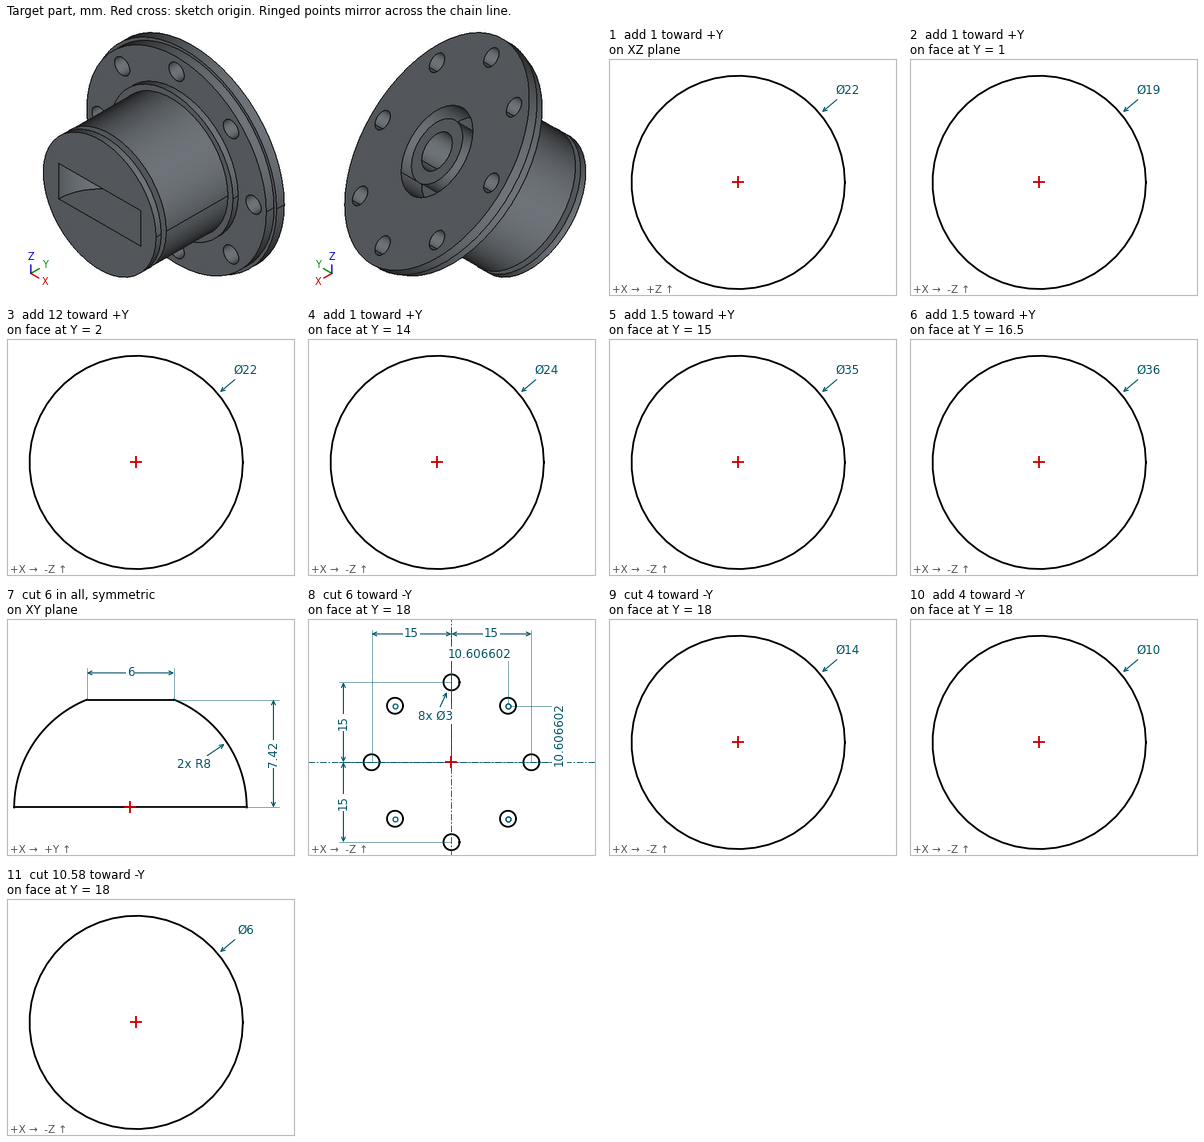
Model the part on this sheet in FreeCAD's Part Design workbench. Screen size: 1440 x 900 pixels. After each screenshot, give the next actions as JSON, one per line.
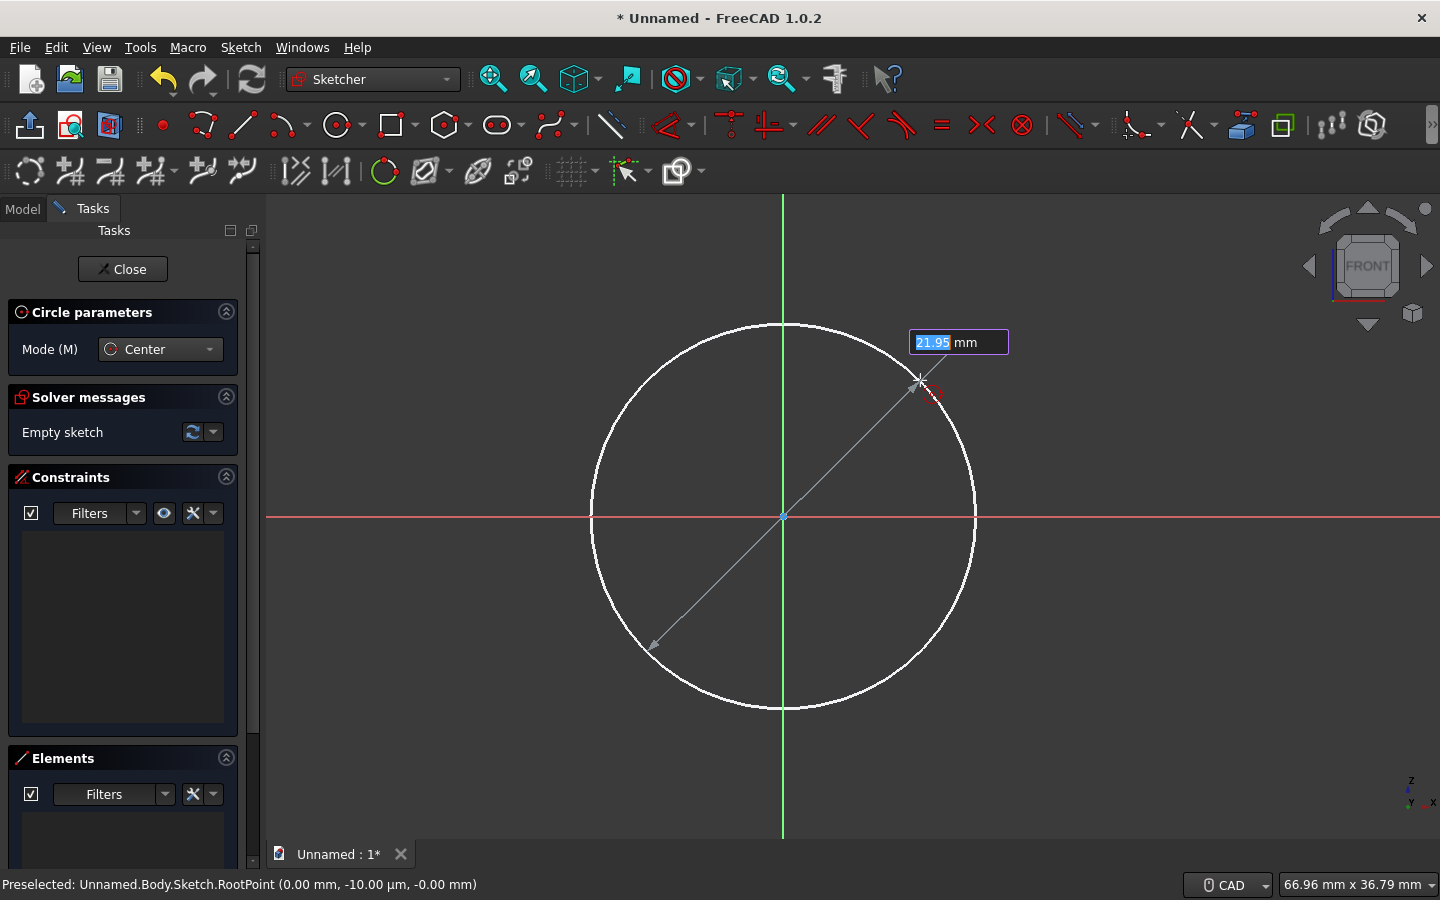
{"action": "type", "text": "22"}
{"action": "key", "text": "Return"}
{"action": "key", "text": "Escape"}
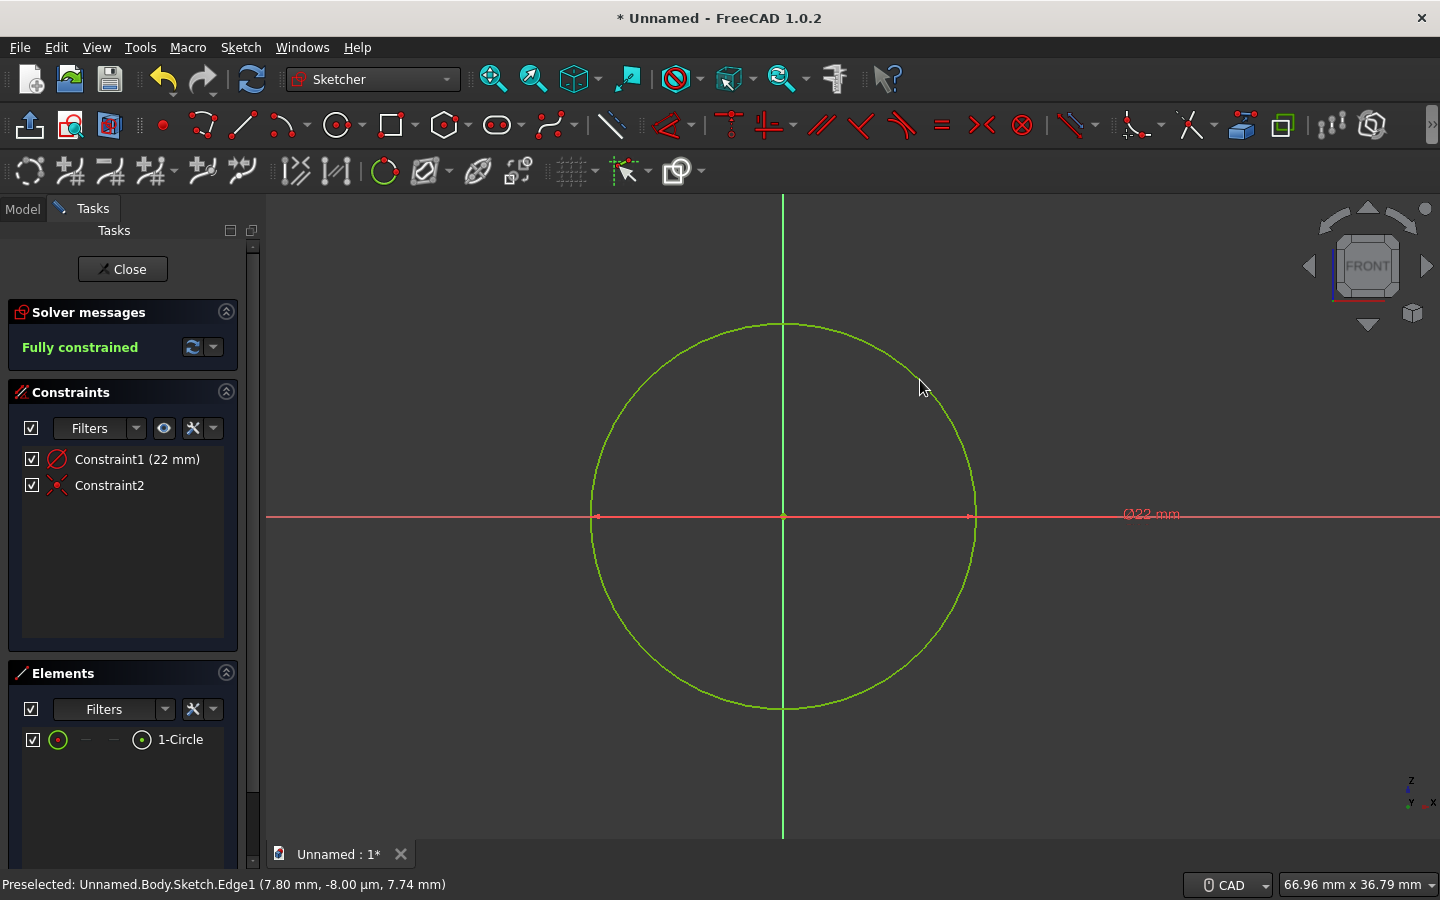
{"action": "left_click", "coordinate": [123, 269]}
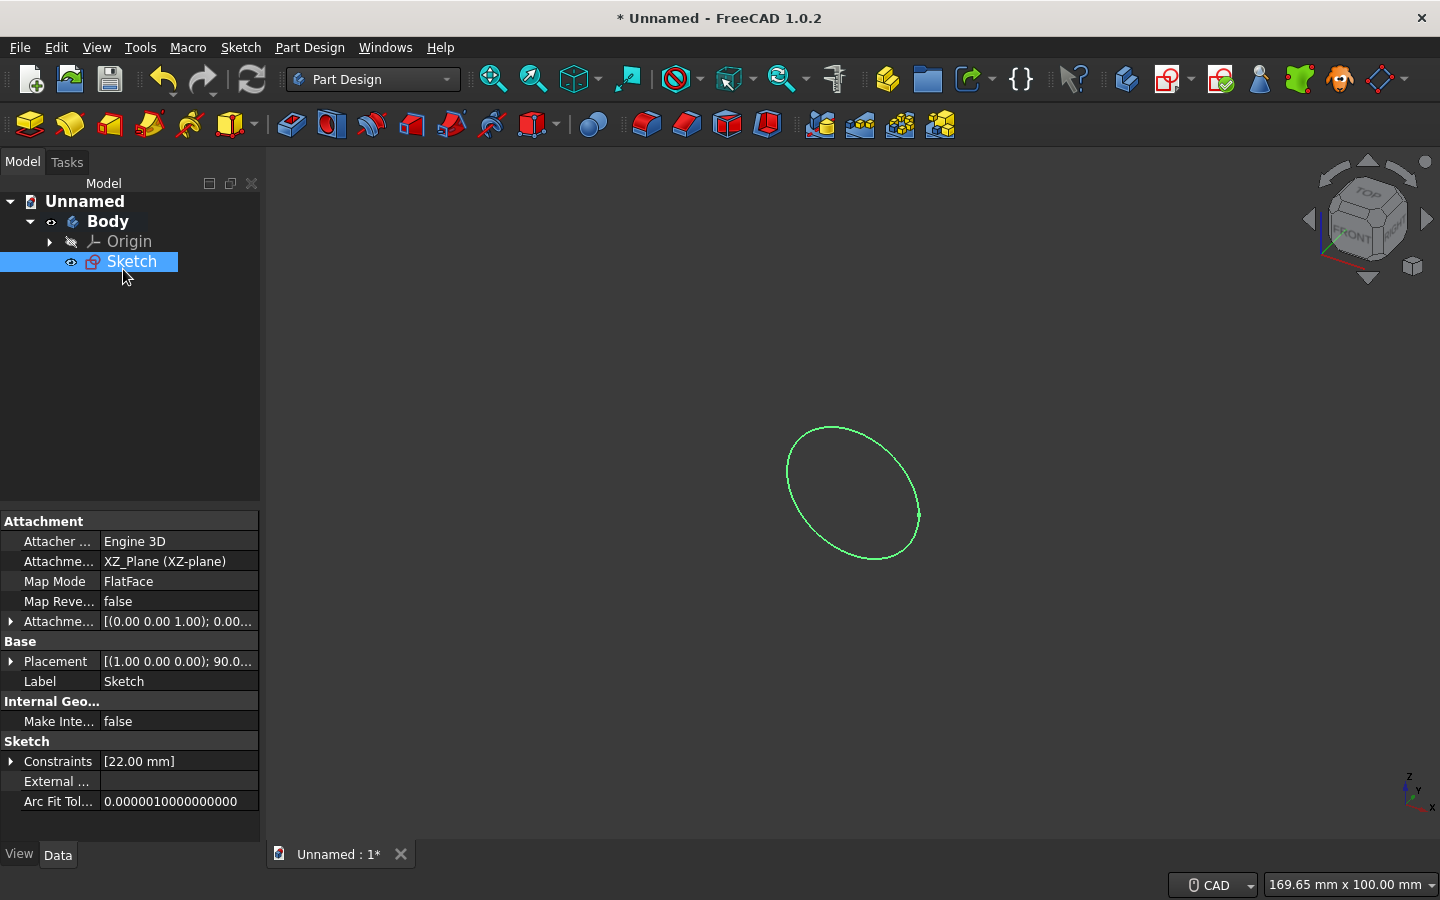
{"action": "left_click", "coordinate": [30, 124]}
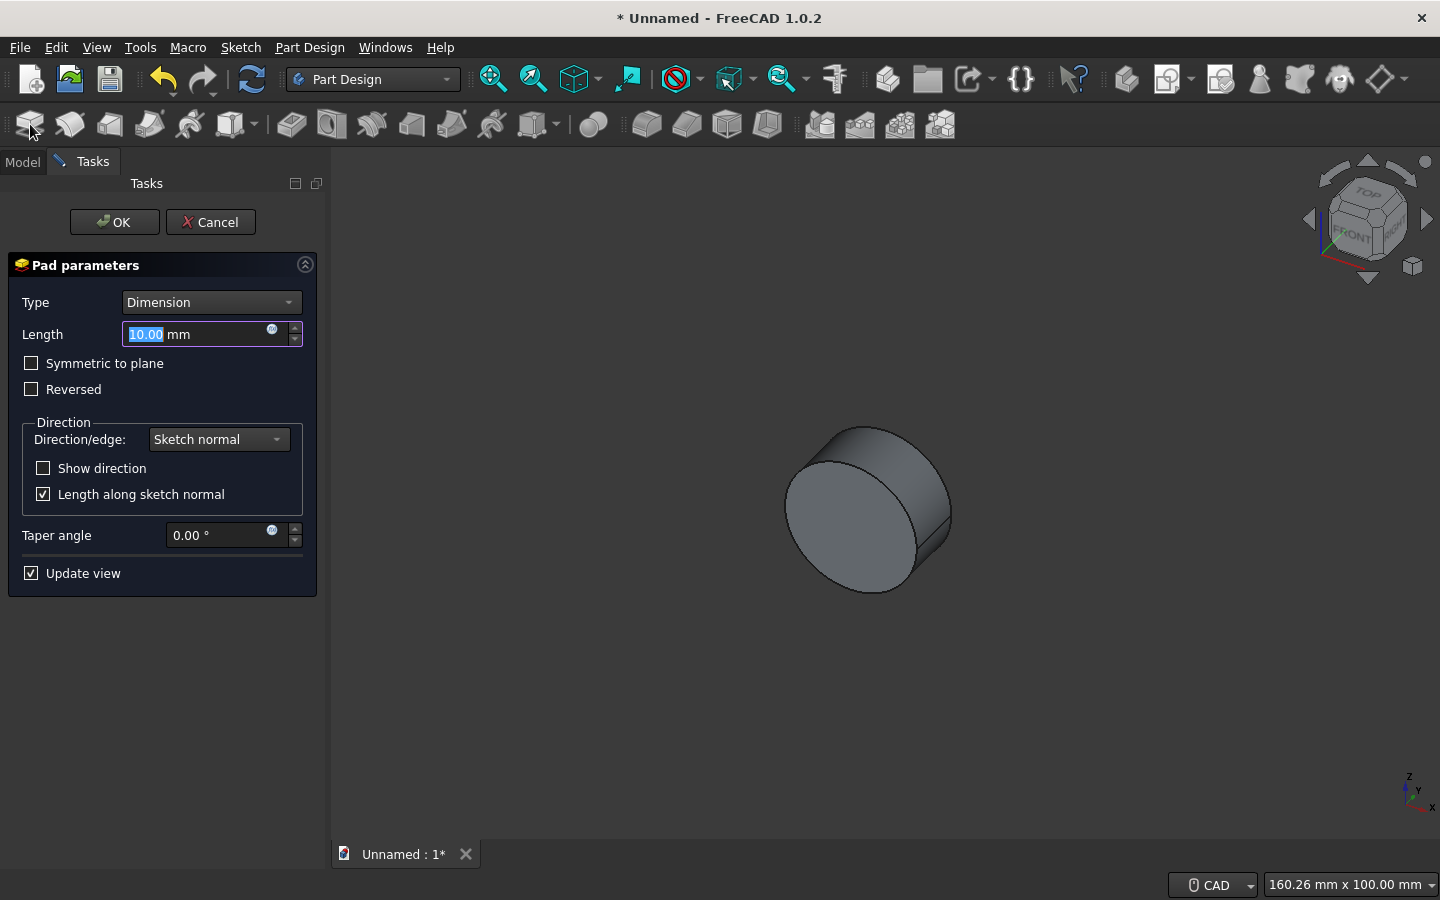
{"action": "type", "text": "1"}
{"action": "key", "text": "Tab"}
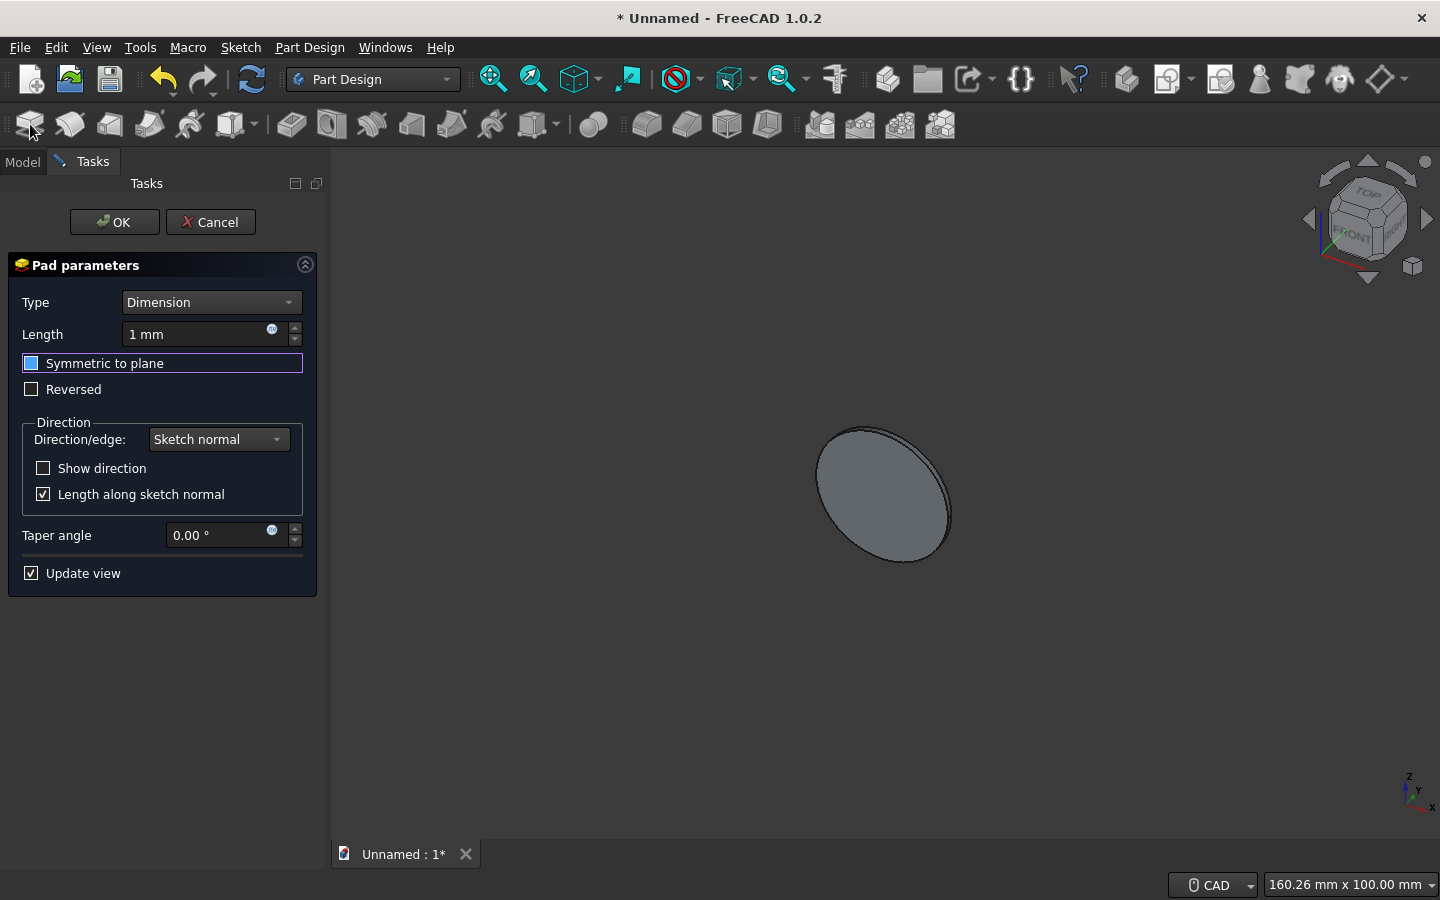
{"action": "left_click", "coordinate": [30, 389]}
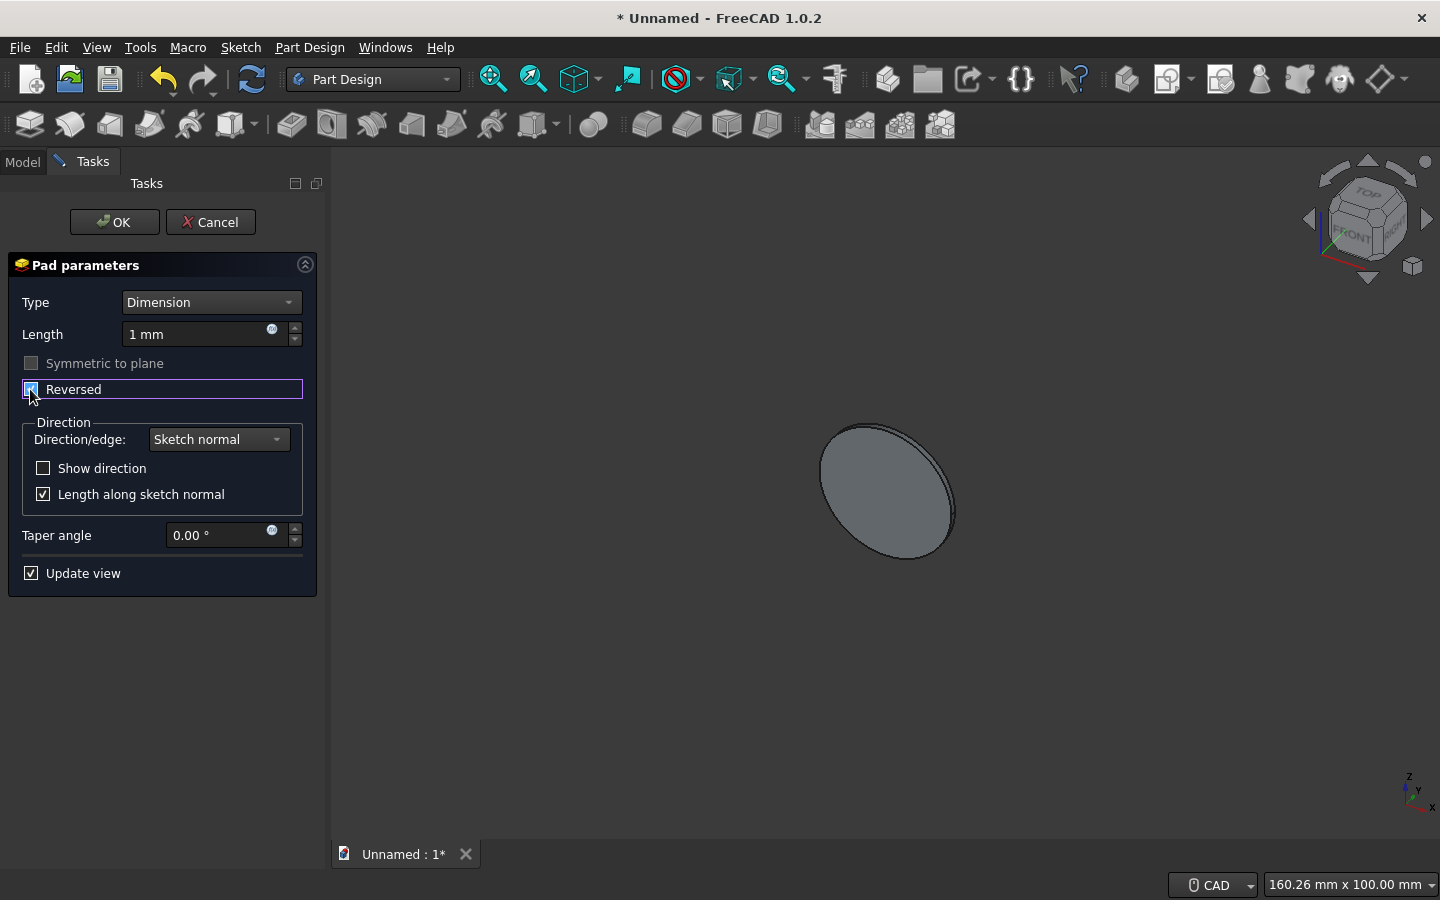
{"action": "left_click", "coordinate": [115, 222]}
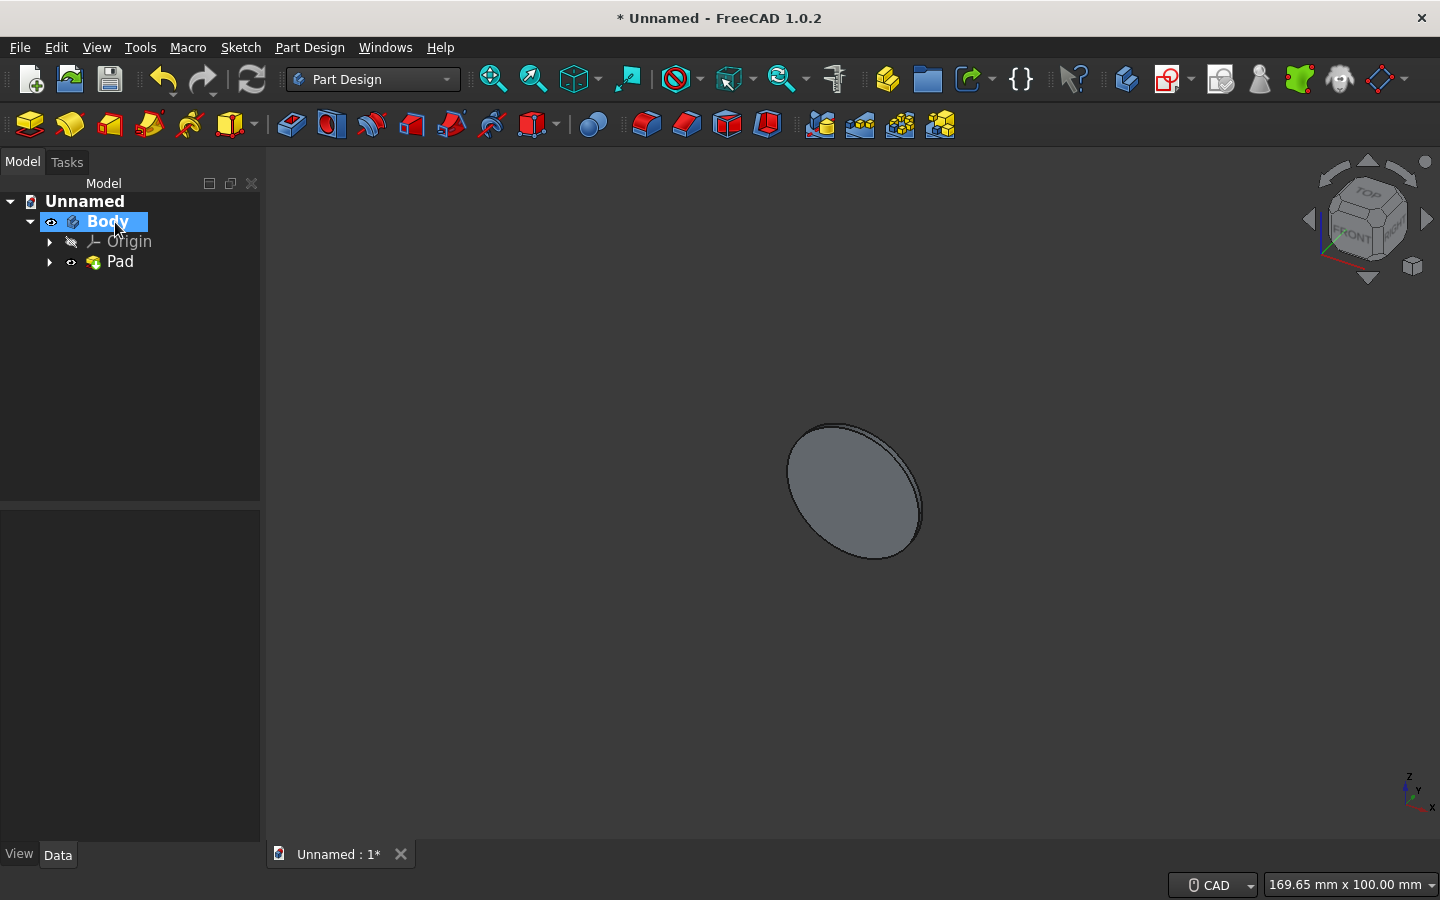
{"action": "left_click", "coordinate": [494, 80]}